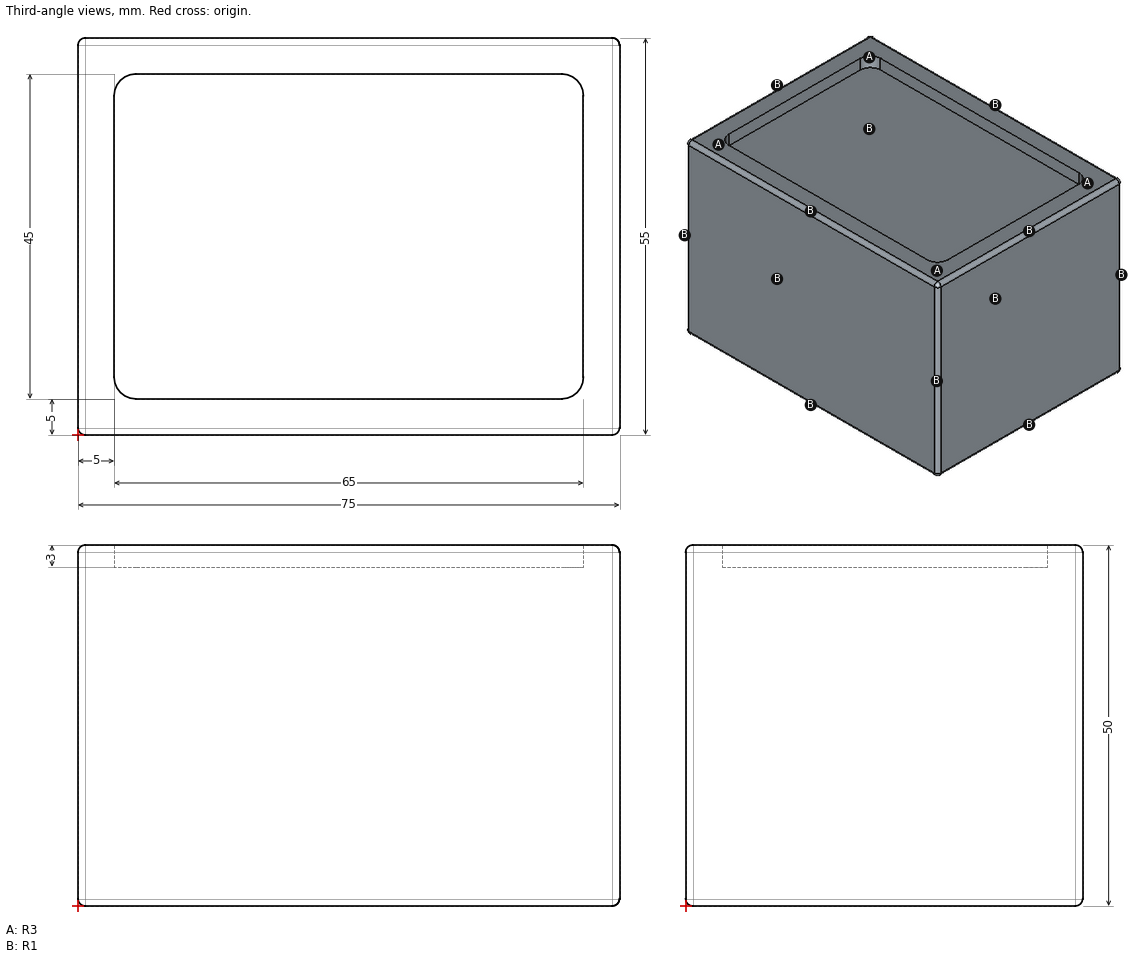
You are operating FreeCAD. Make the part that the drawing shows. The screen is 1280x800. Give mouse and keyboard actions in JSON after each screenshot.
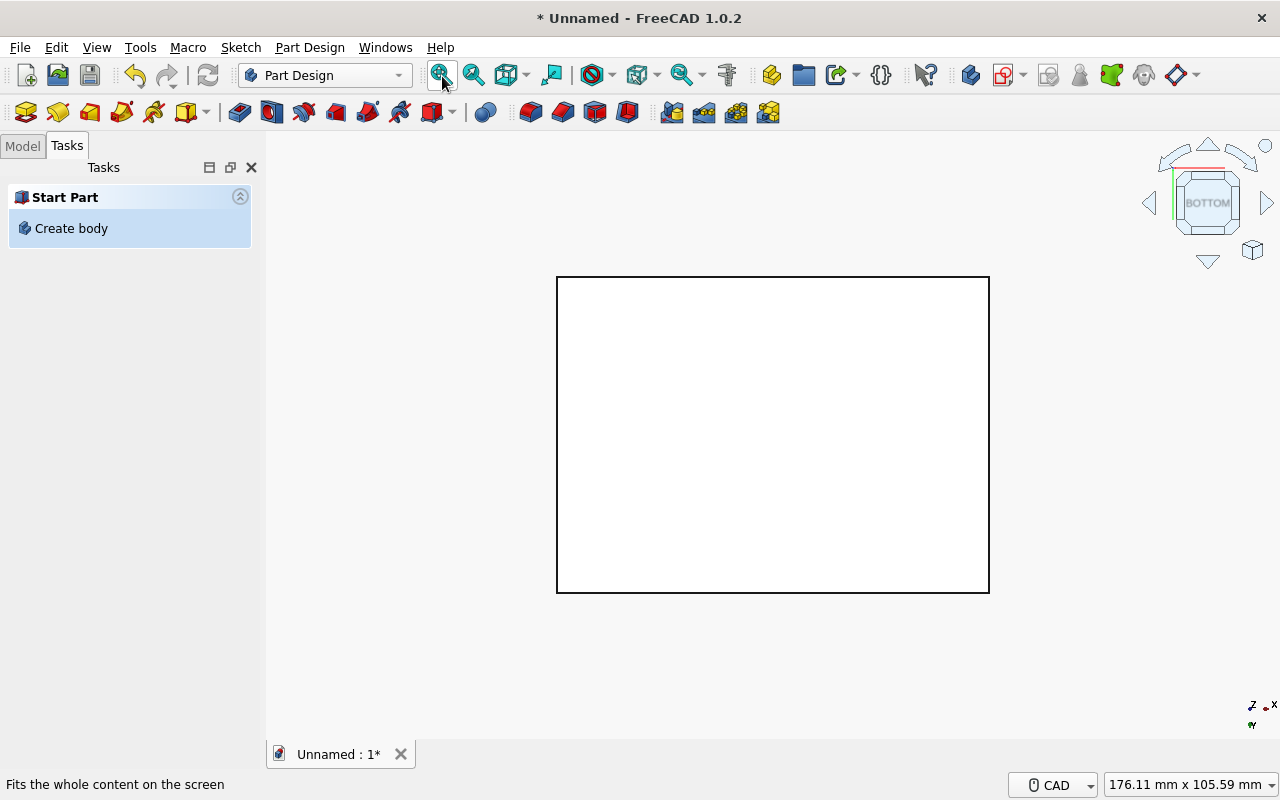
{"action": "key", "text": "4"}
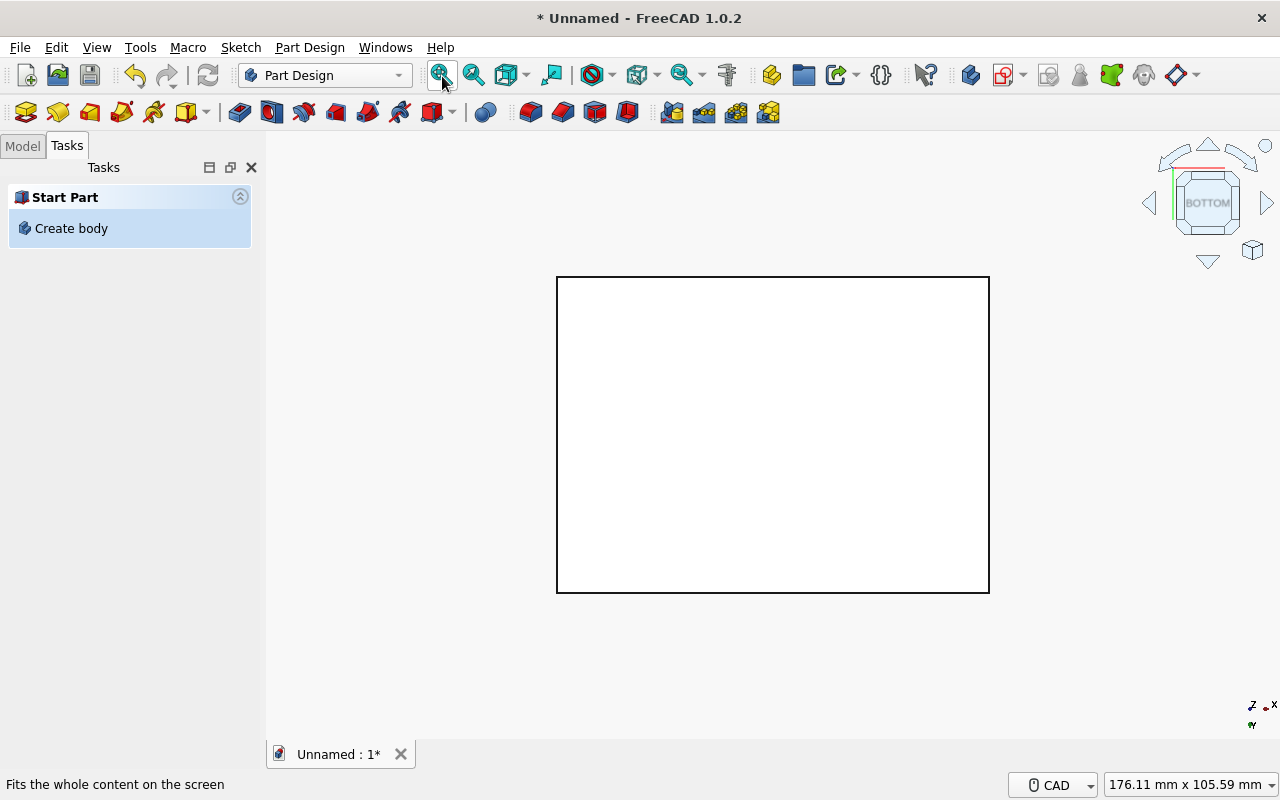
{"action": "scroll", "coordinate": [960, 299], "scroll_direction": "up", "scroll_amount": 5}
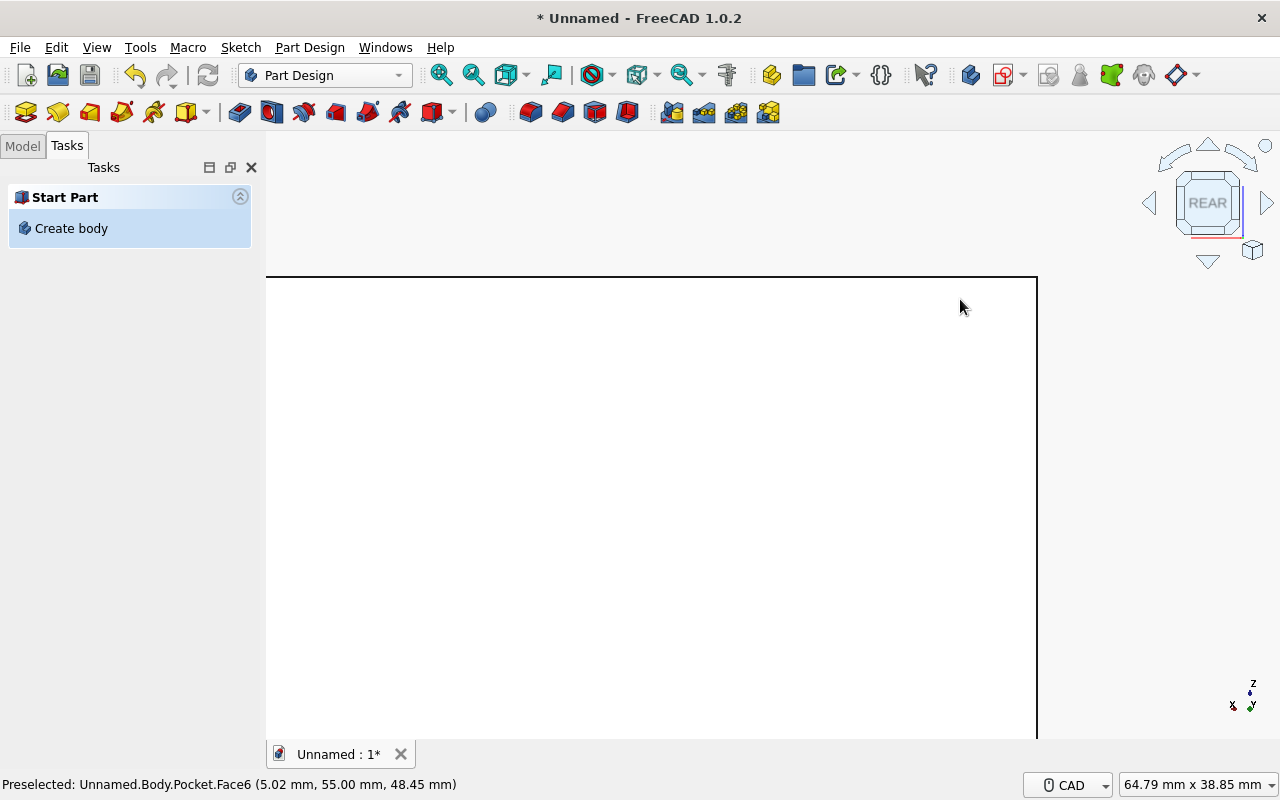
{"action": "left_click", "coordinate": [442, 76]}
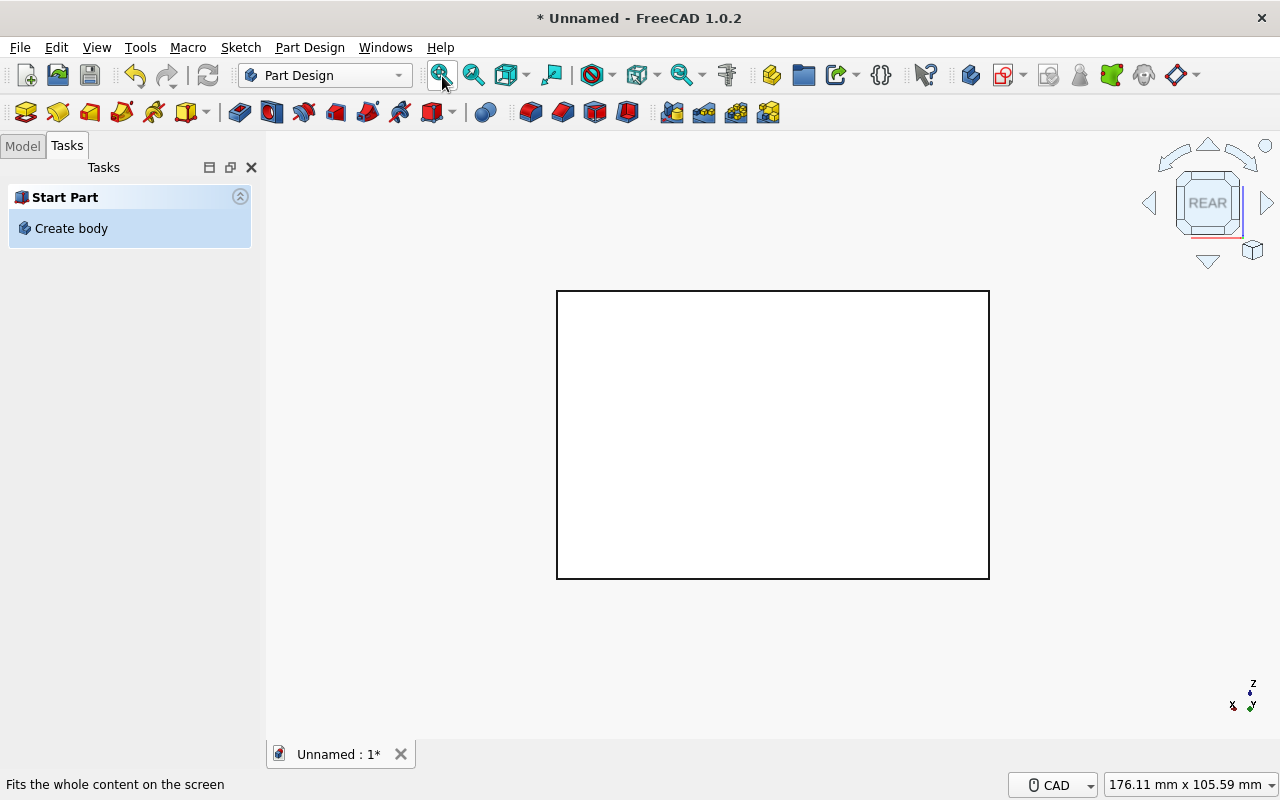
{"action": "key", "text": "6"}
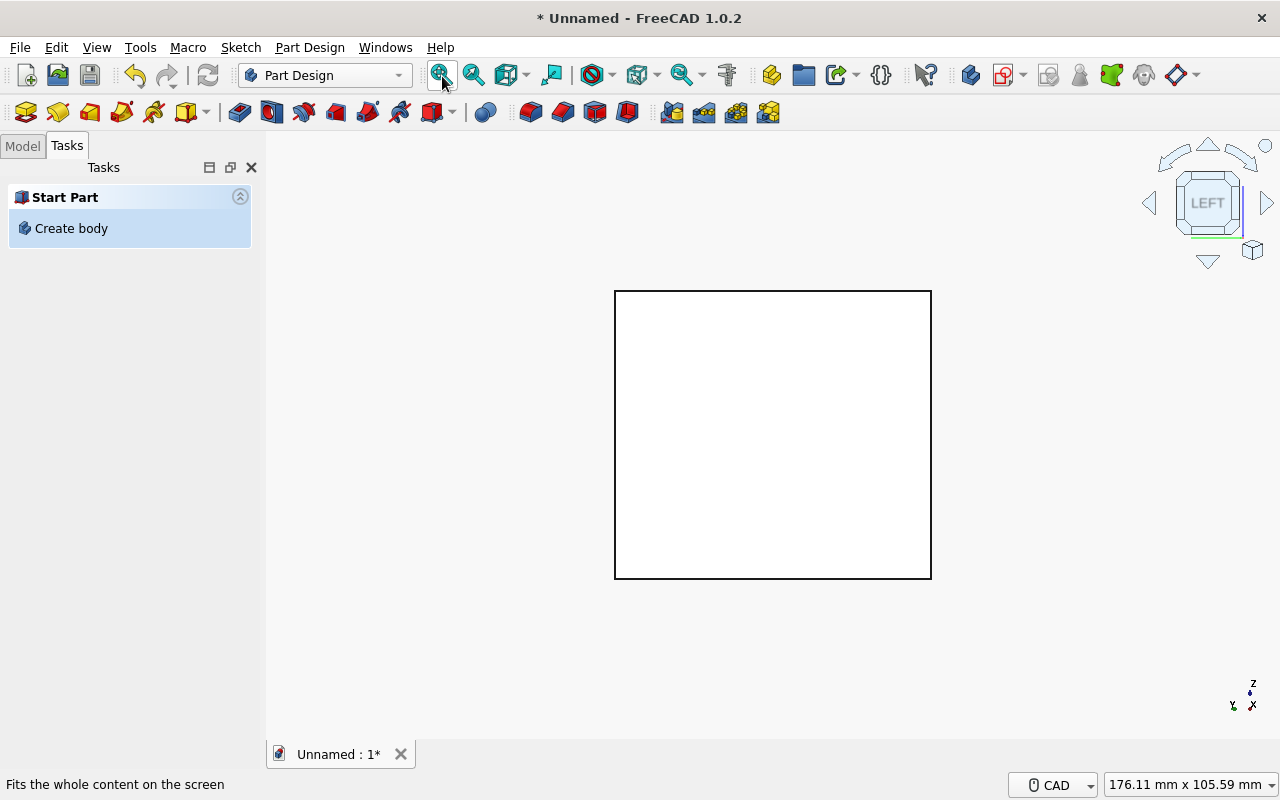
{"action": "scroll", "coordinate": [903, 299], "scroll_direction": "up", "scroll_amount": 5}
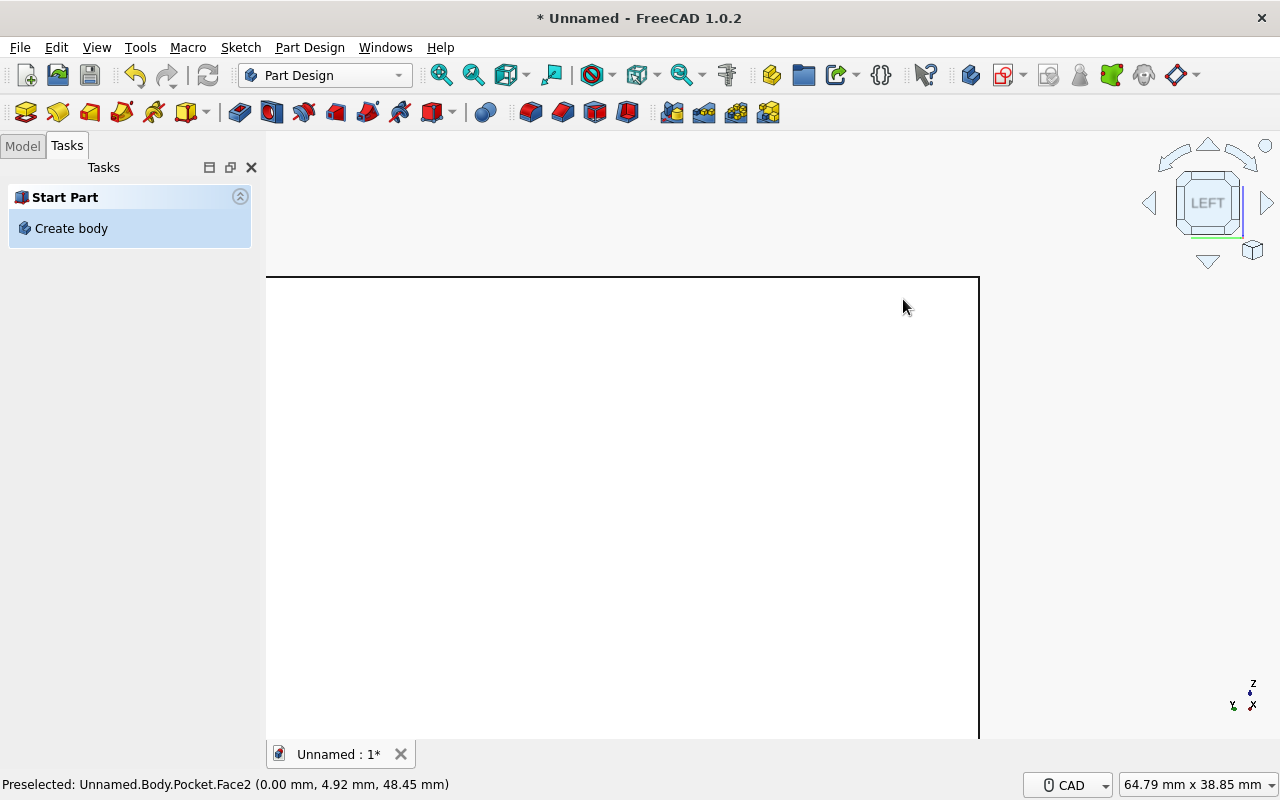
{"action": "left_click", "coordinate": [442, 76]}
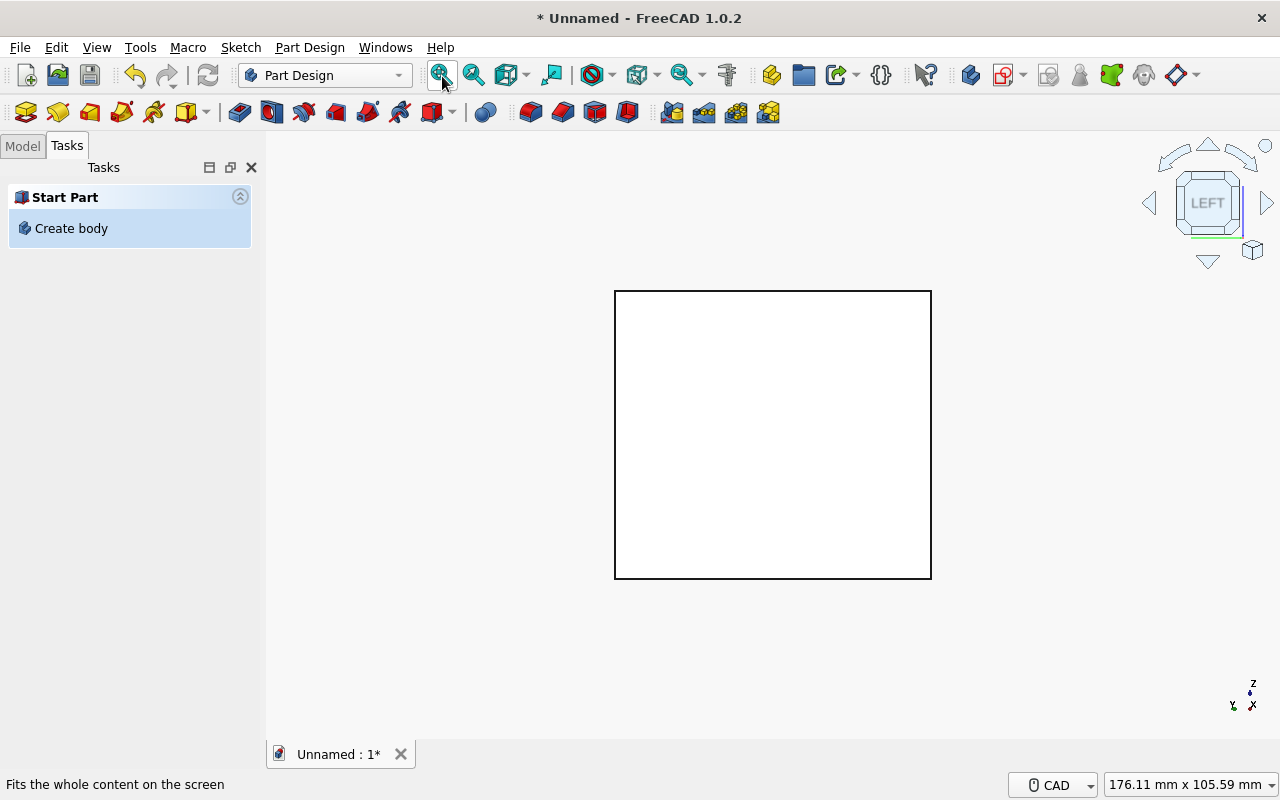
{"action": "key", "text": "v 3"}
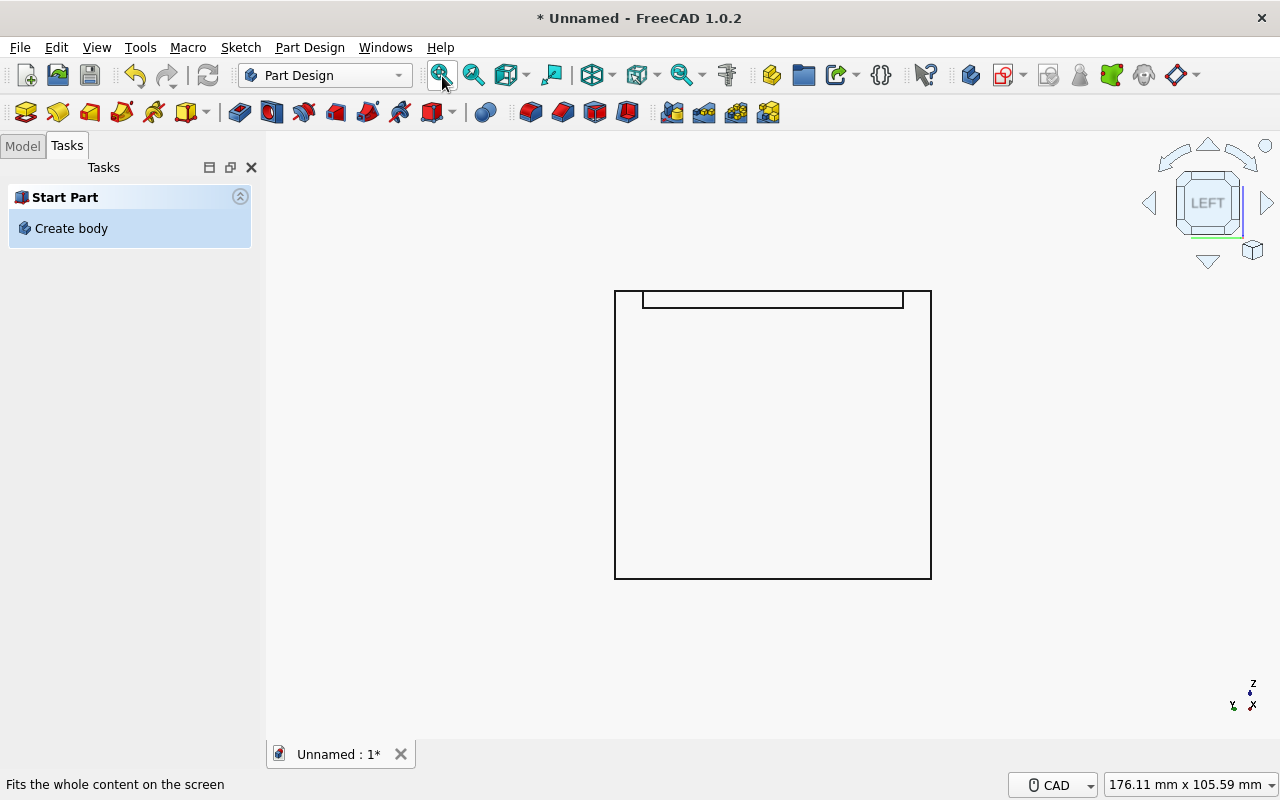
{"action": "key", "text": "0"}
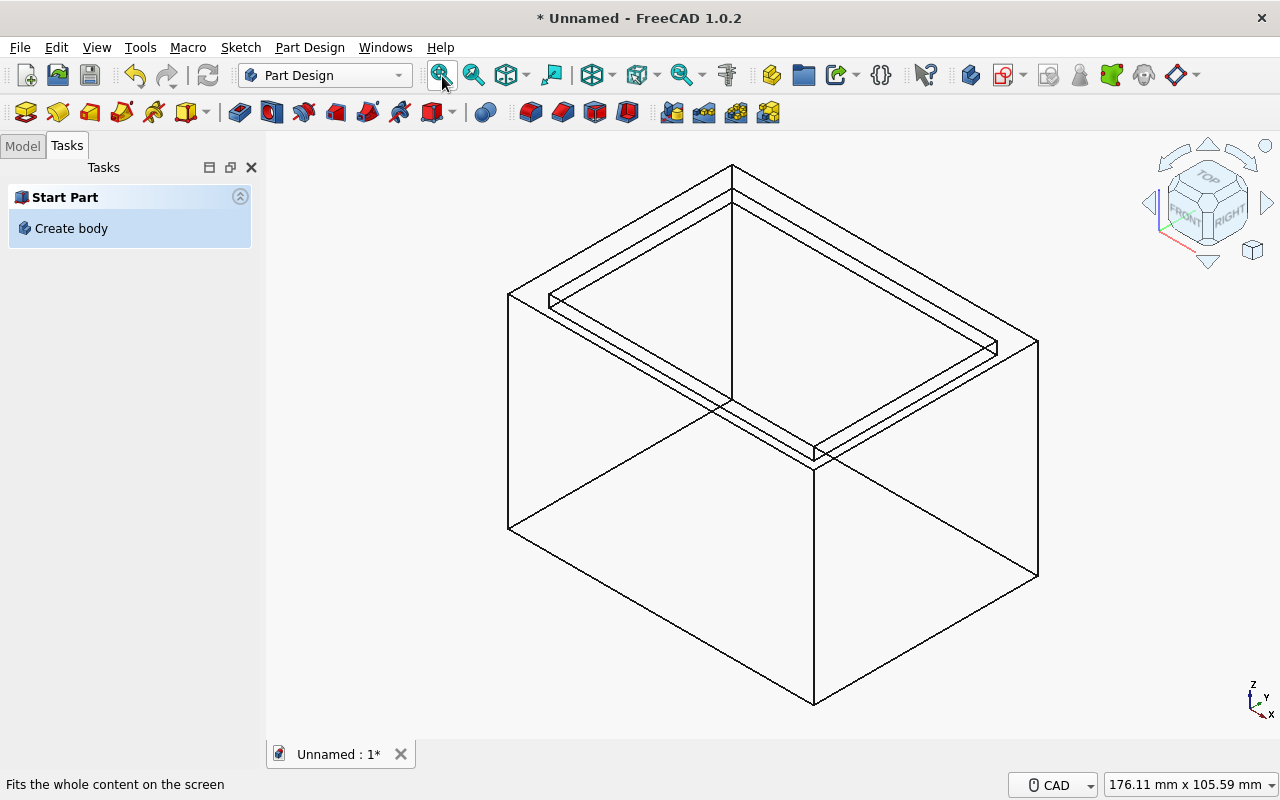
{"action": "left_click", "coordinate": [549, 301]}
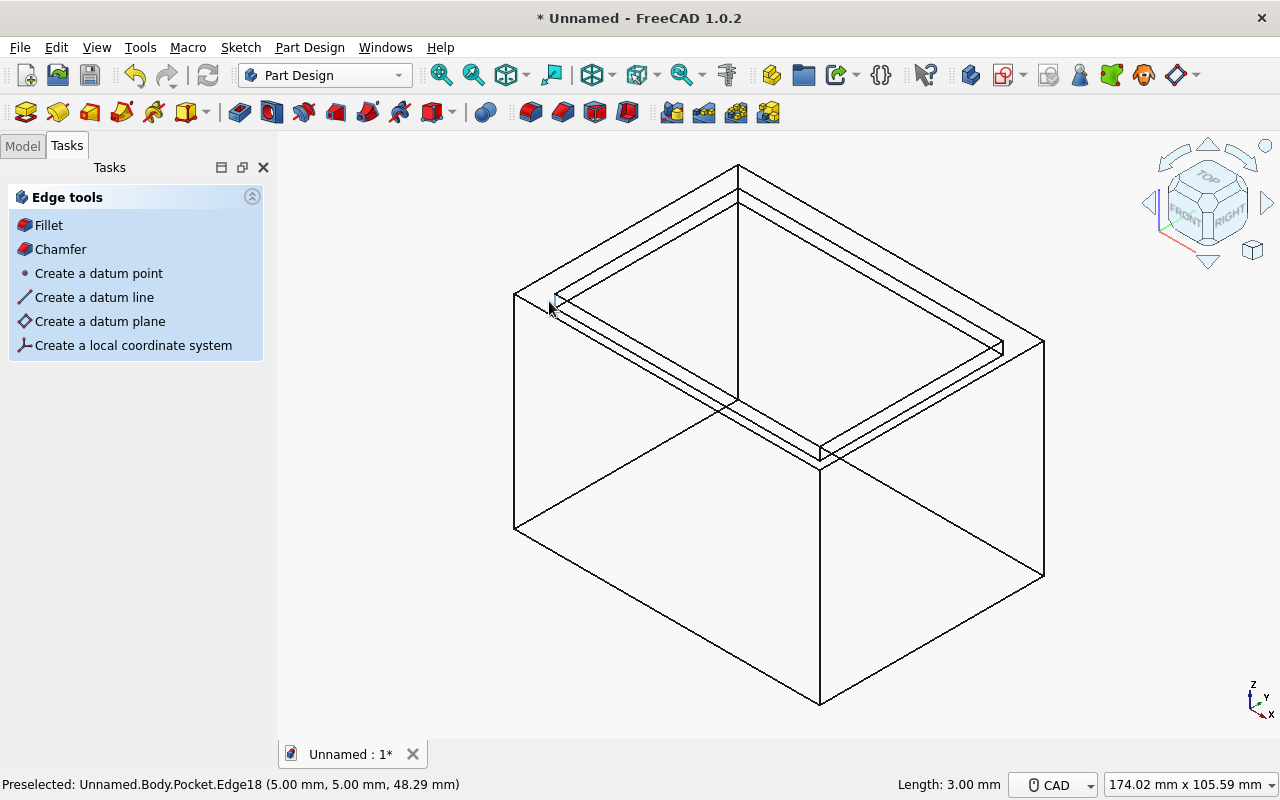
{"action": "left_click", "coordinate": [738, 196], "text": "ctrl"}